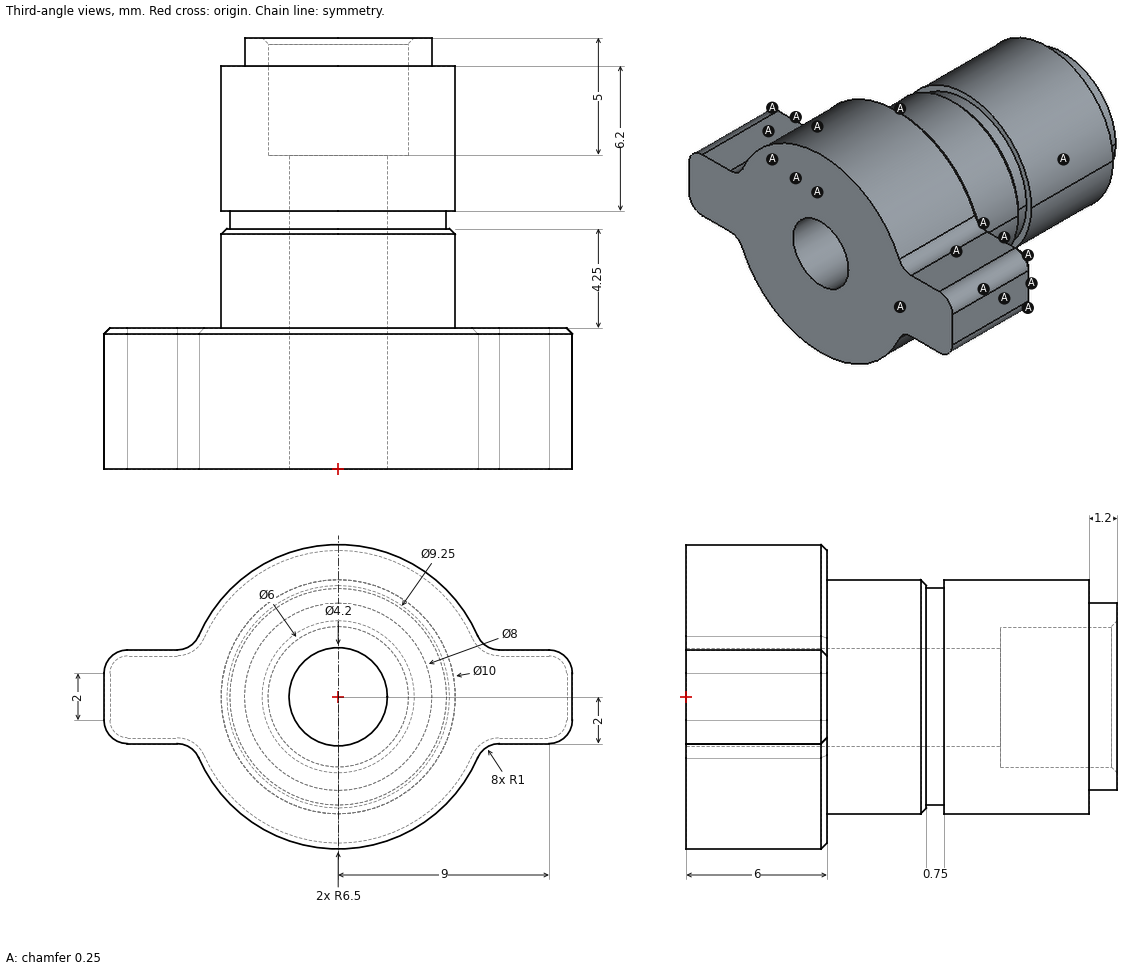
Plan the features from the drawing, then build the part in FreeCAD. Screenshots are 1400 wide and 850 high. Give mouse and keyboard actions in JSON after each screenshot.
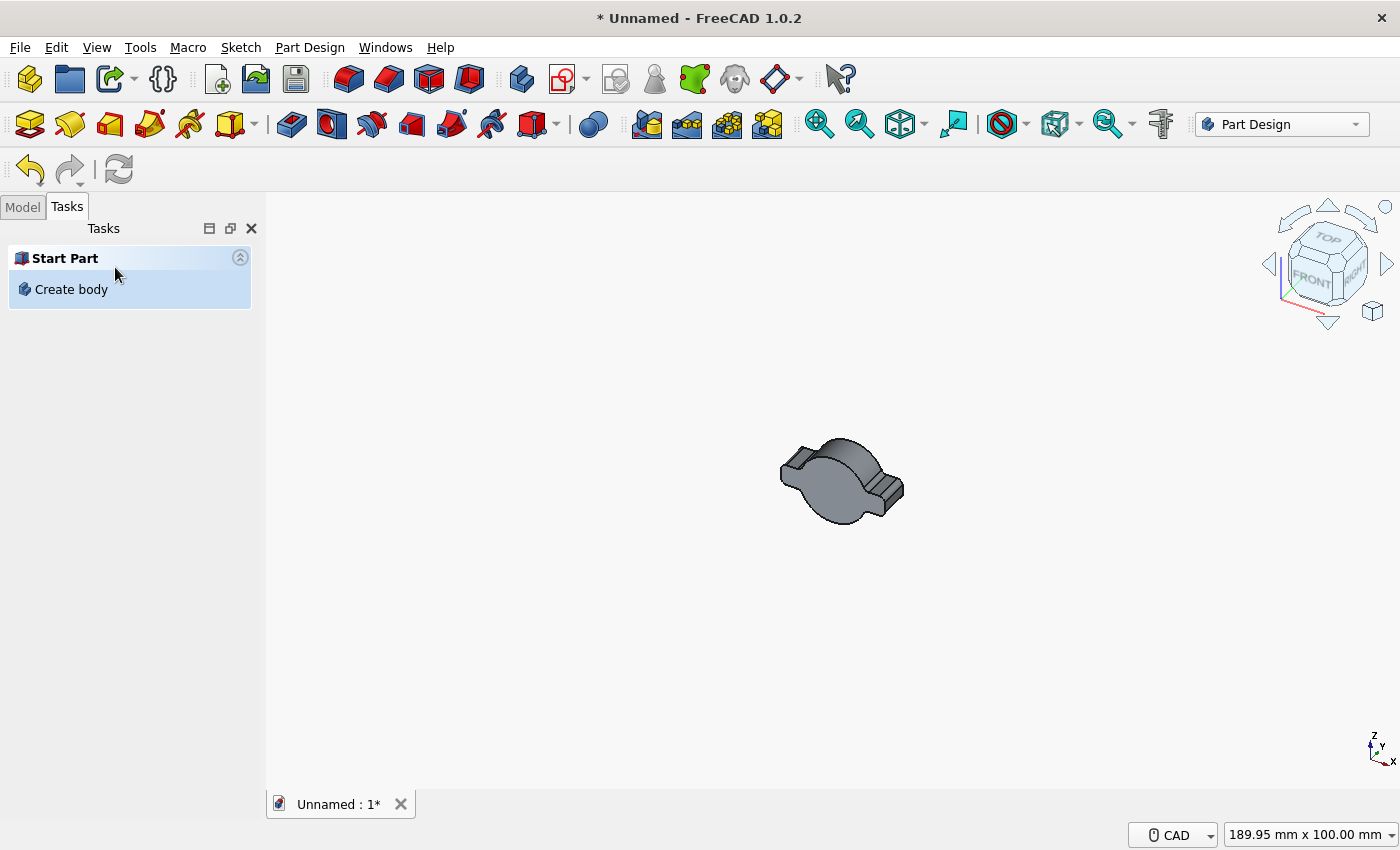
{"action": "left_click", "coordinate": [820, 124]}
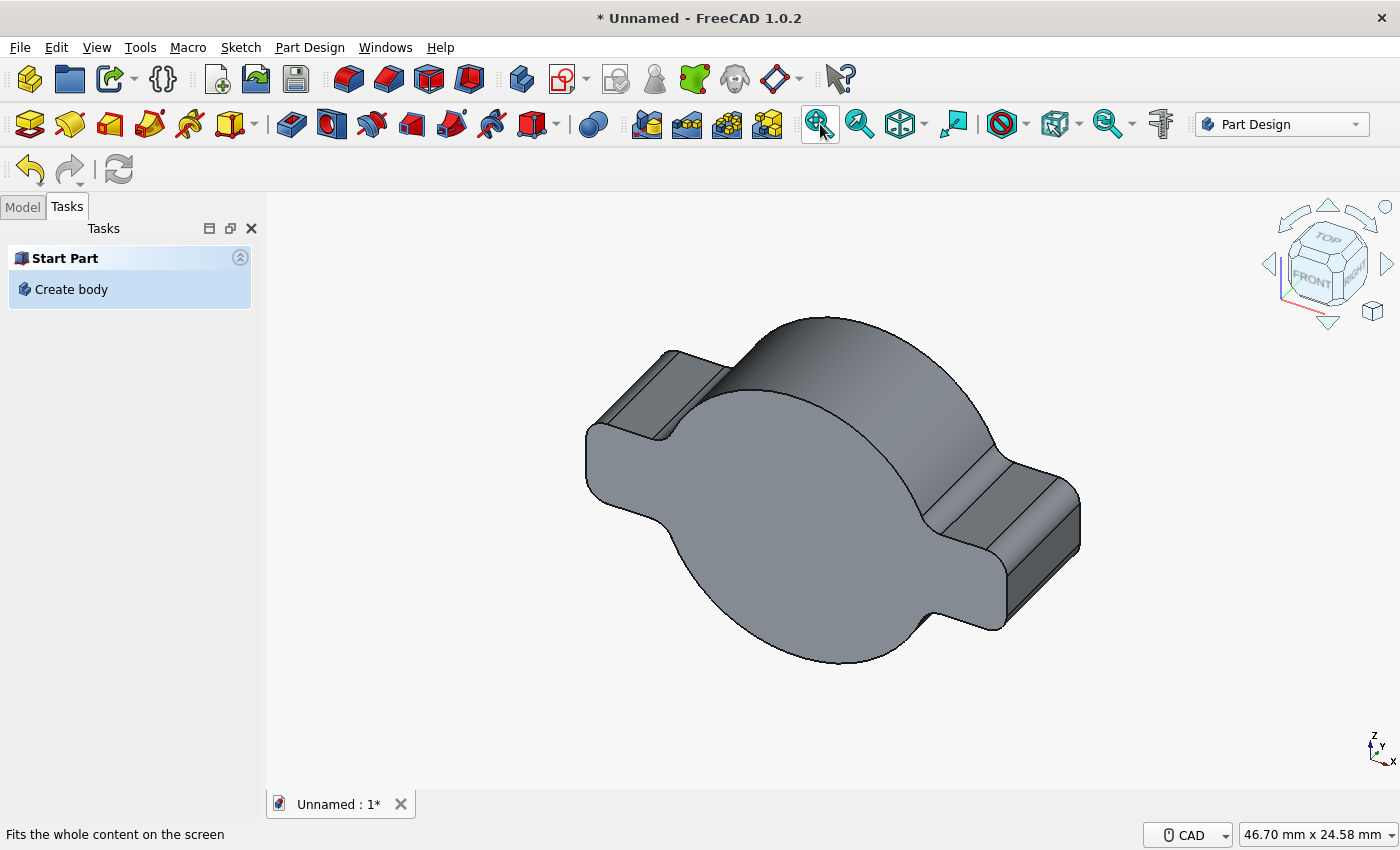
{"action": "key", "text": "4"}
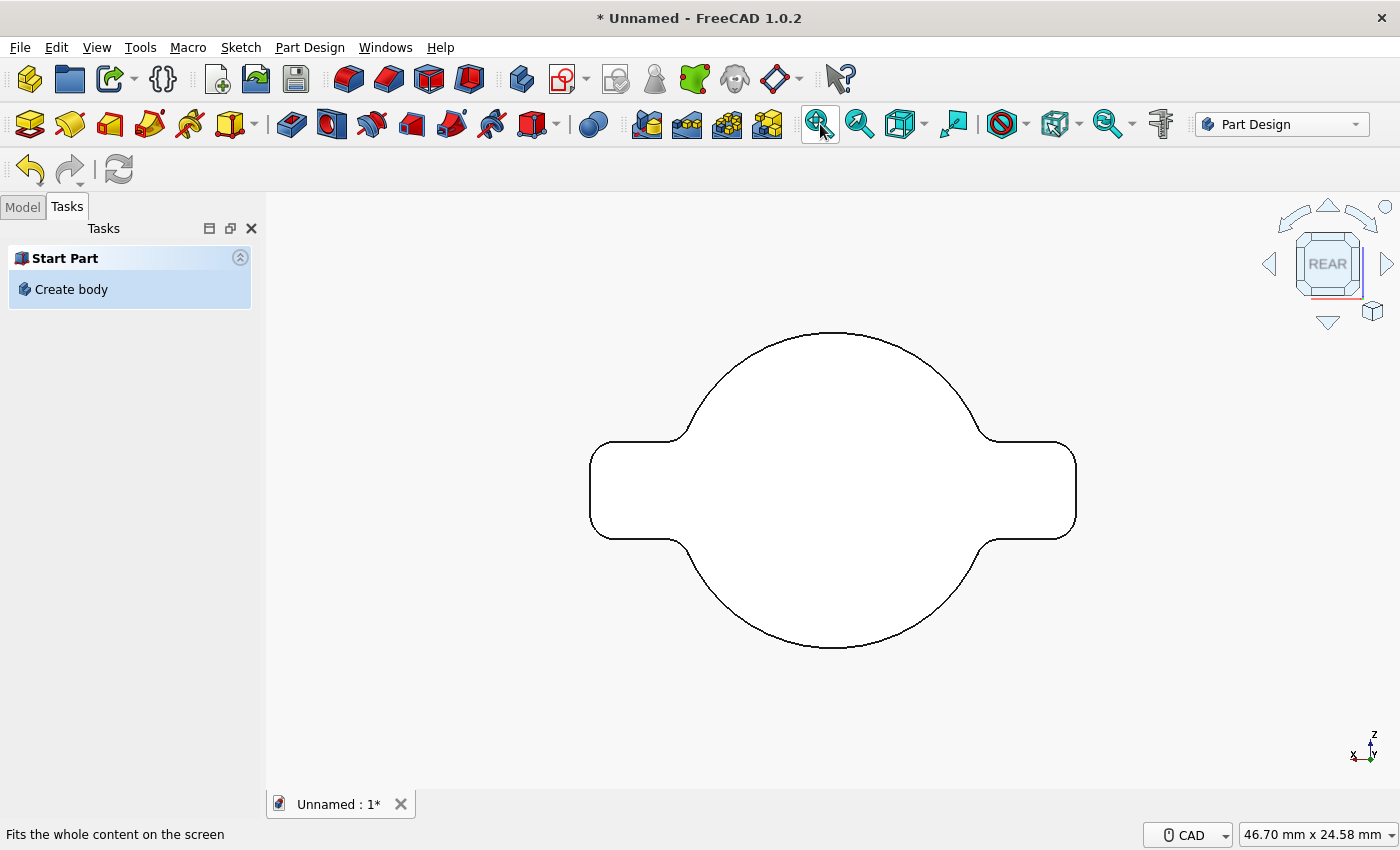
{"action": "left_click", "coordinate": [833, 490]}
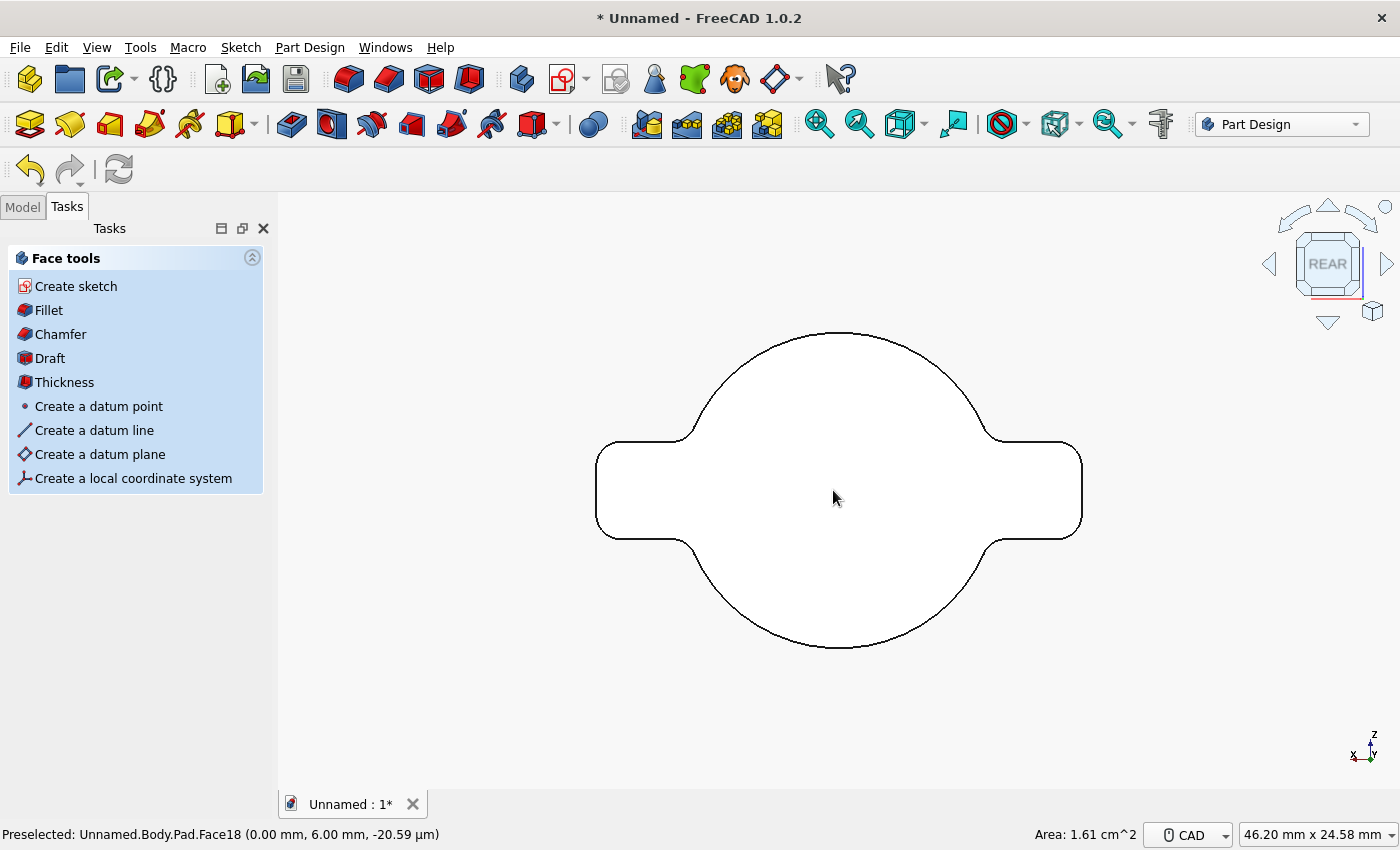
{"action": "left_click", "coordinate": [562, 80]}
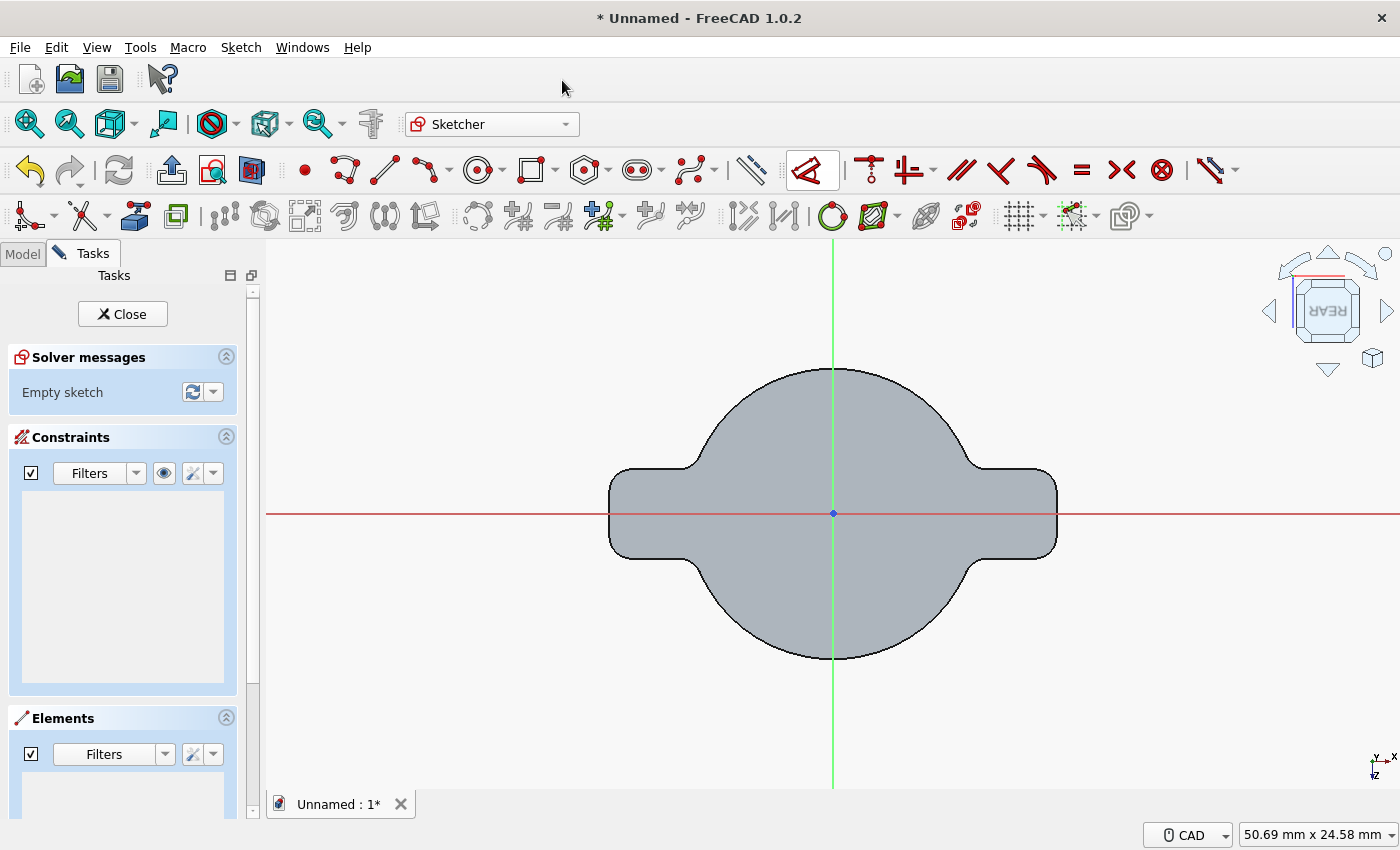
{"action": "scroll", "coordinate": [972, 514], "scroll_direction": "up", "scroll_amount": 2}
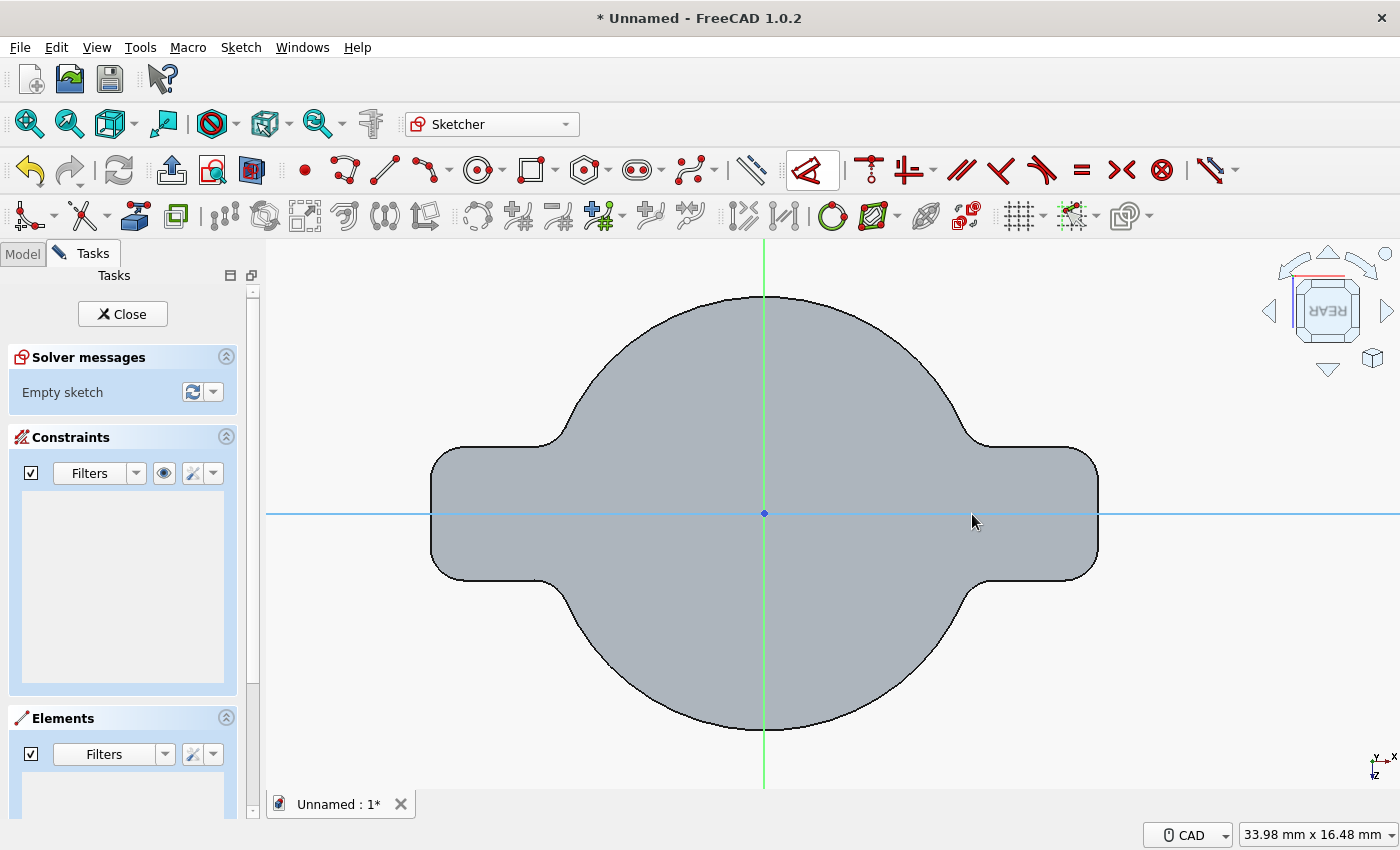
{"action": "left_click", "coordinate": [478, 170]}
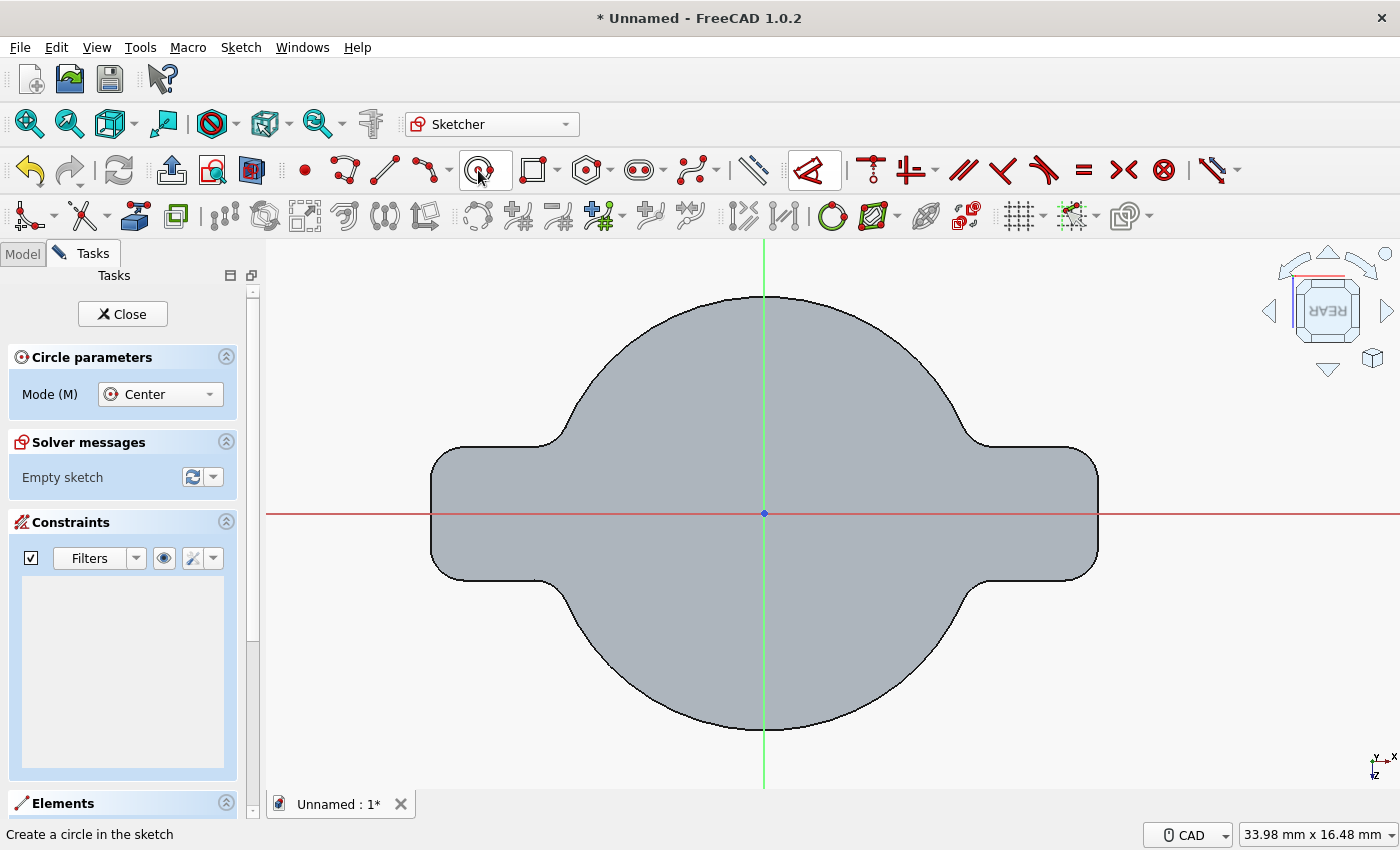
{"action": "left_click", "coordinate": [764, 514]}
{"action": "mouse_move", "coordinate": [882, 396]}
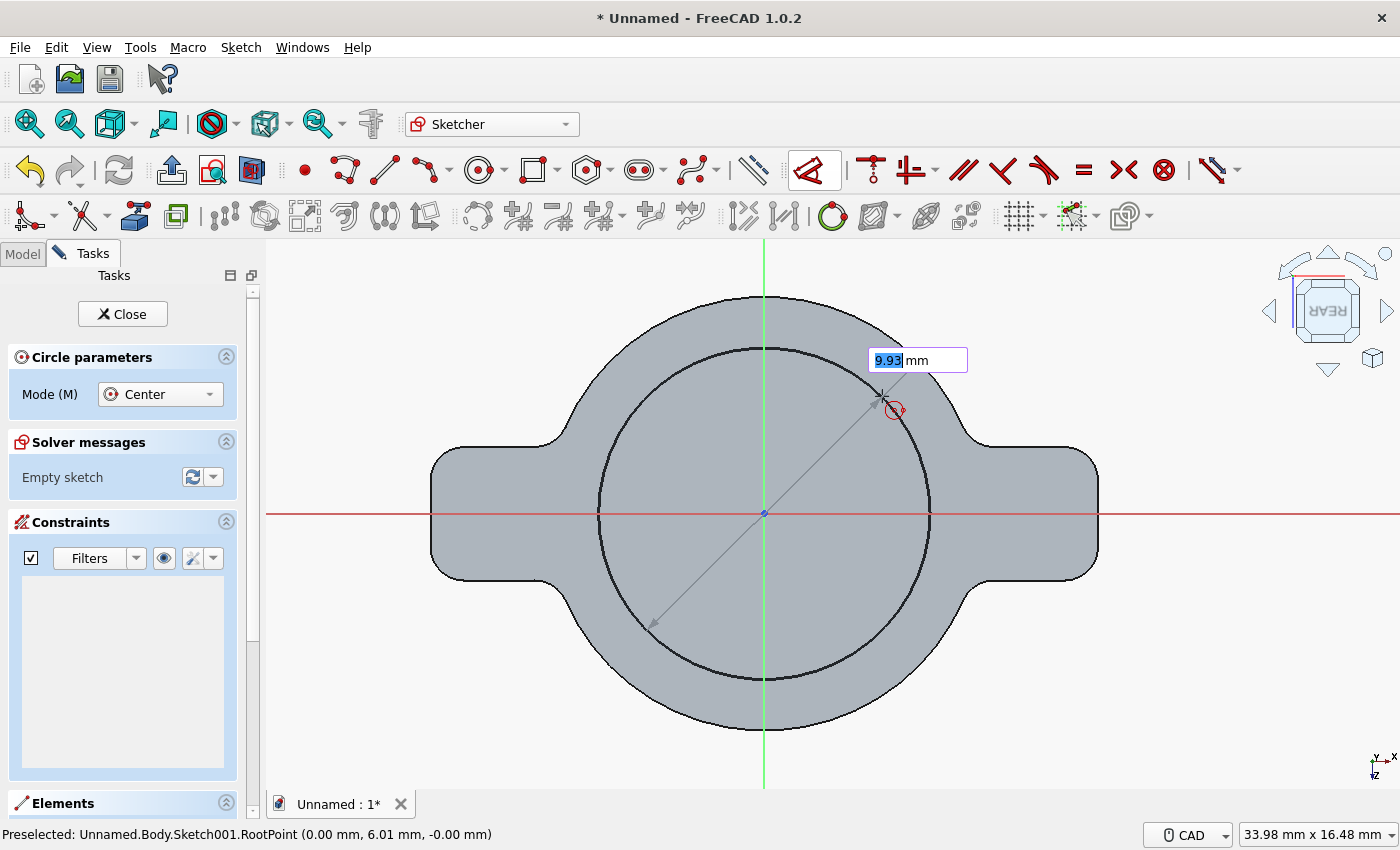
{"action": "type", "text": "10"}
{"action": "key", "text": "Return"}
{"action": "key", "text": "Escape"}